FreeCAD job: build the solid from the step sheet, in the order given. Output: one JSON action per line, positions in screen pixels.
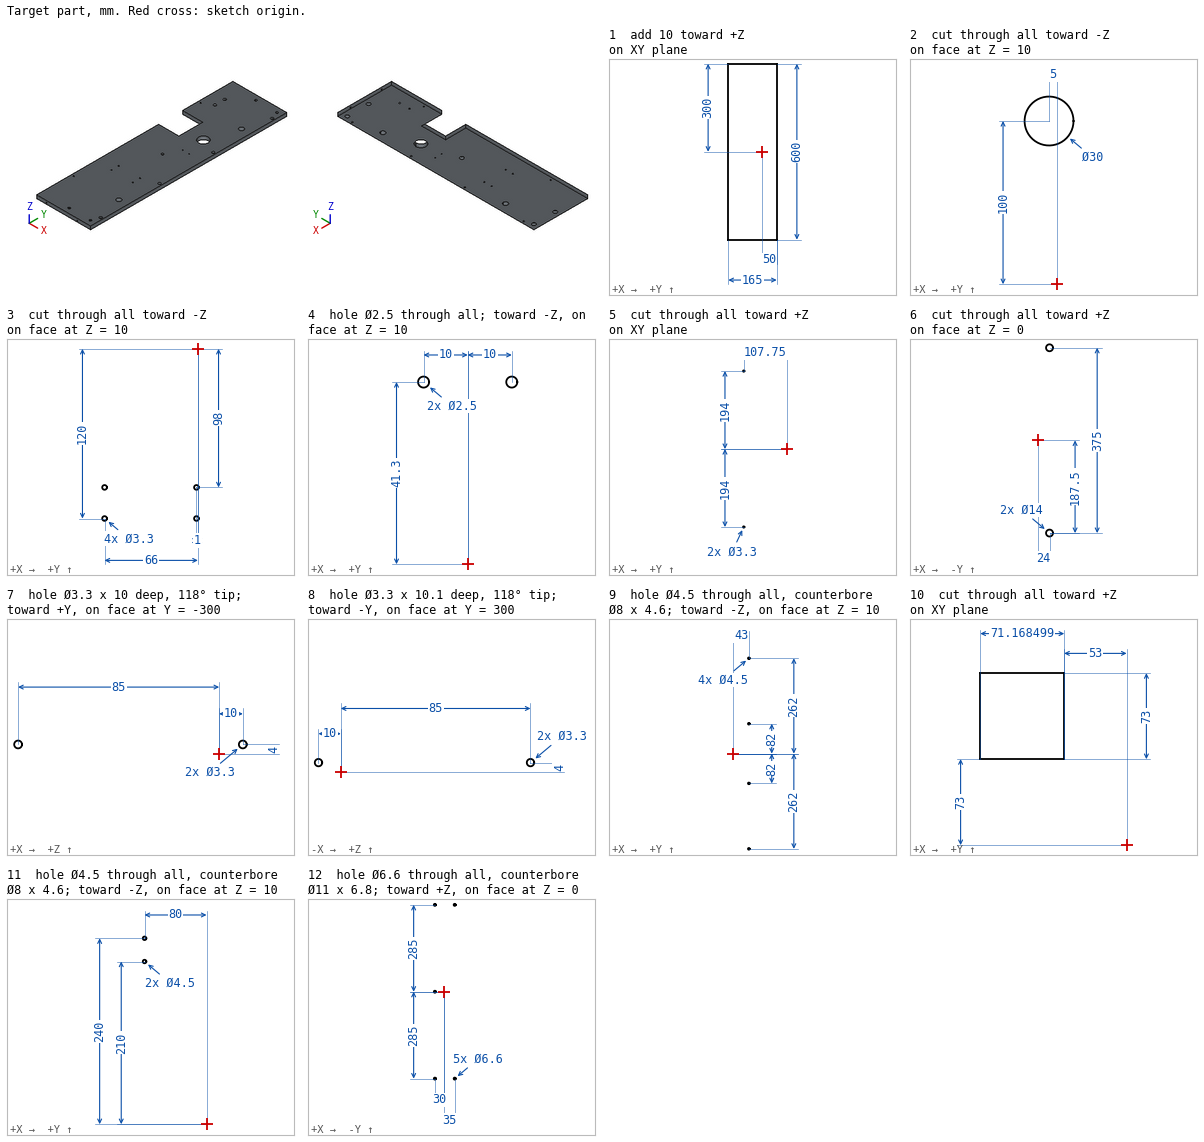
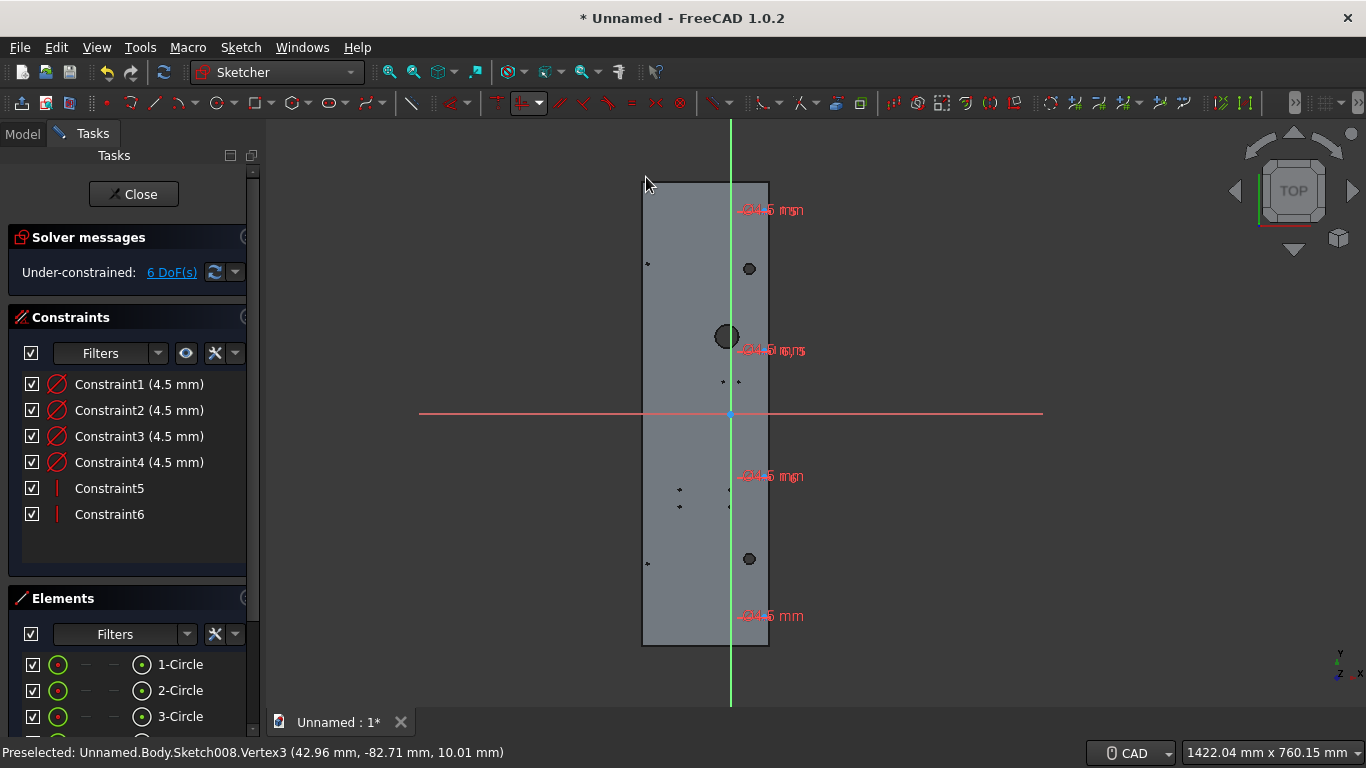
{"action": "left_click", "coordinate": [764, 478]}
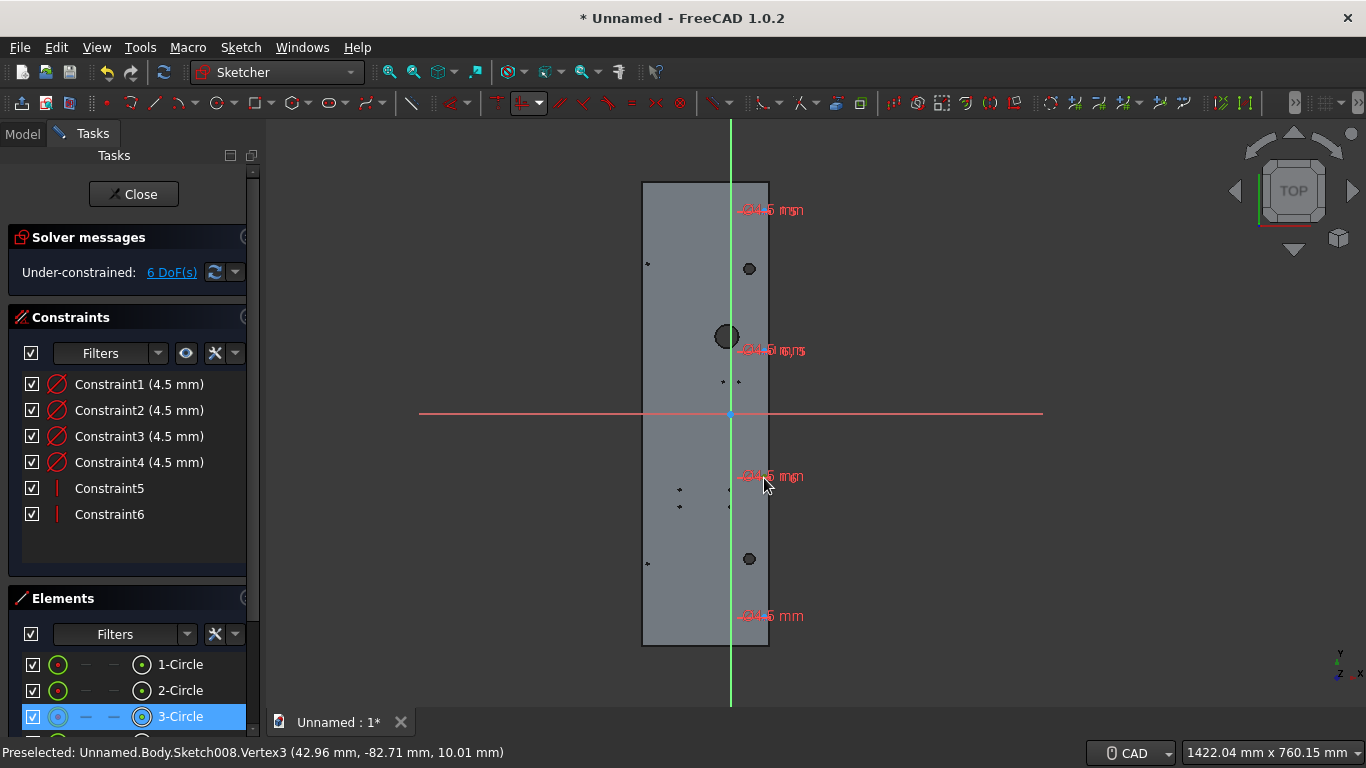
{"action": "left_click", "coordinate": [764, 618]}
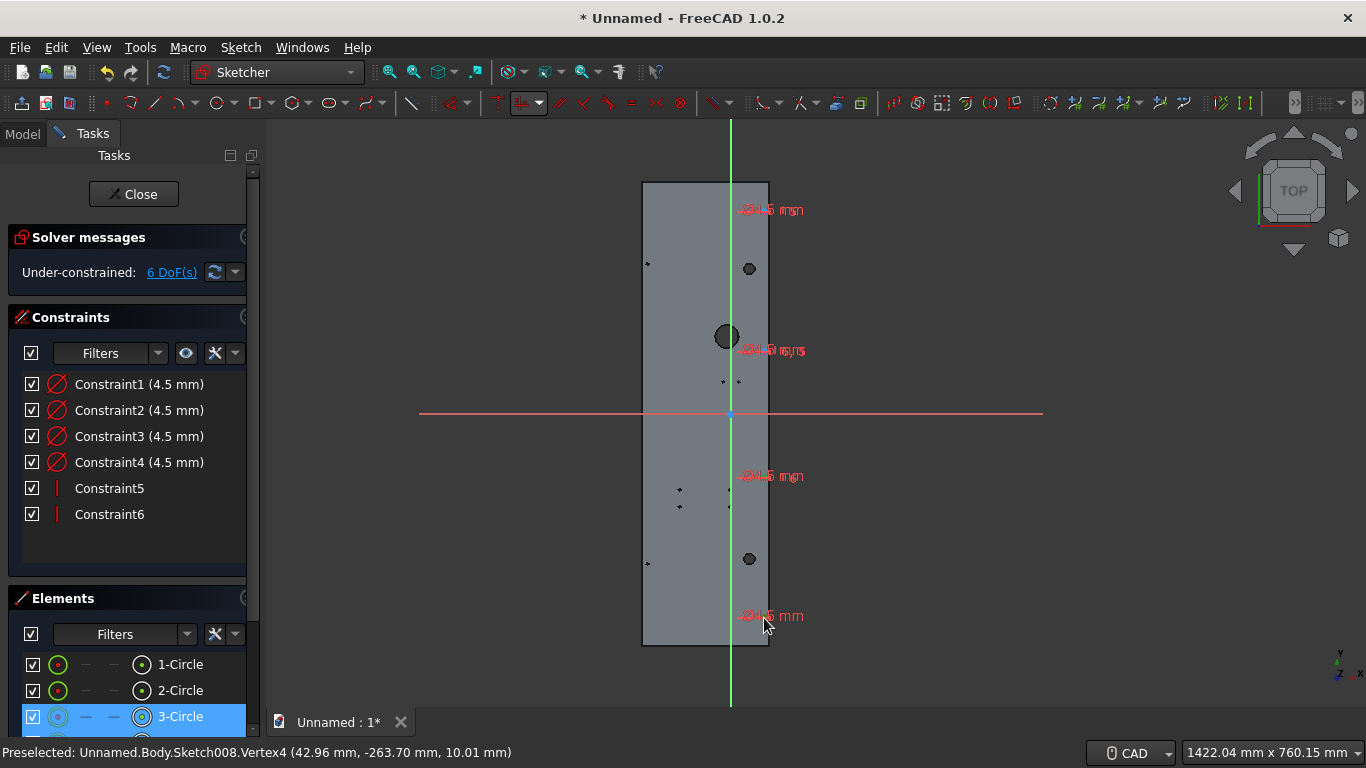
{"action": "left_click", "coordinate": [542, 104]}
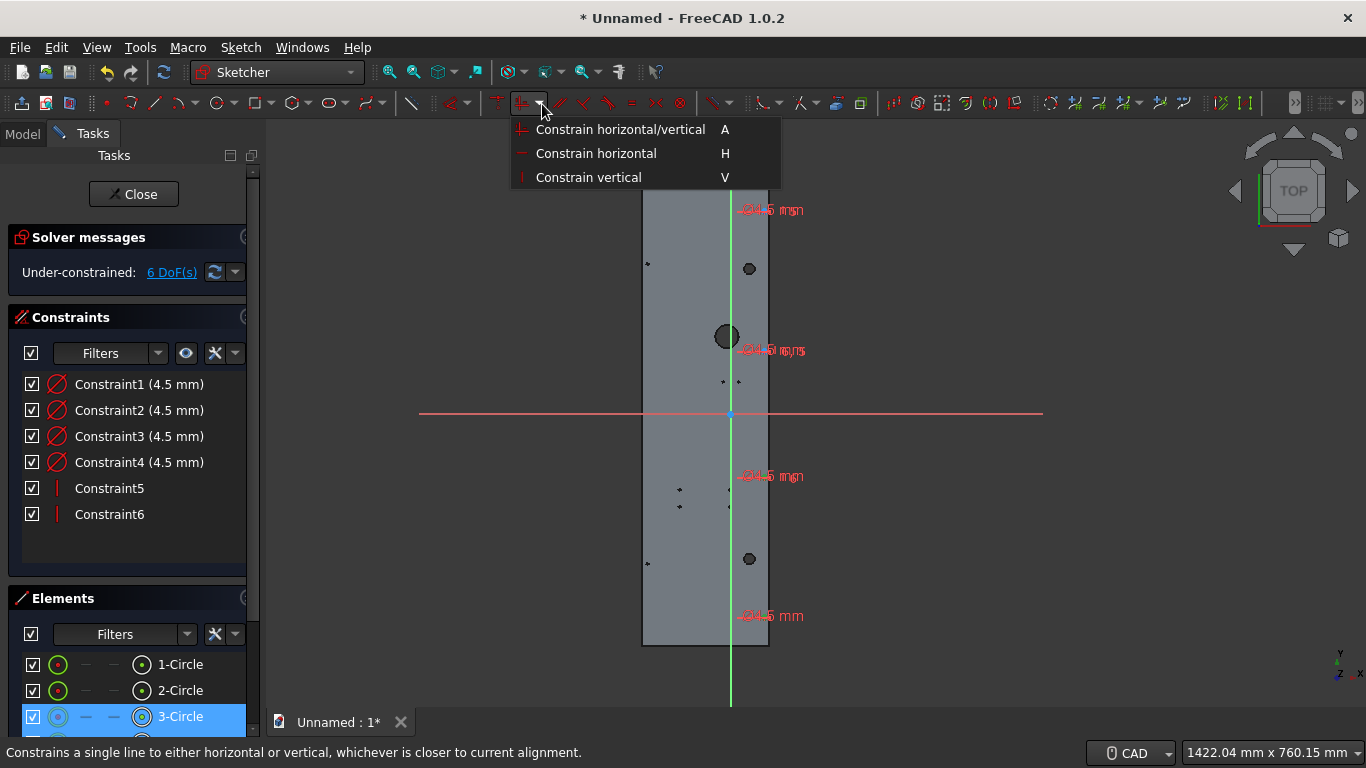
{"action": "left_click", "coordinate": [646, 177]}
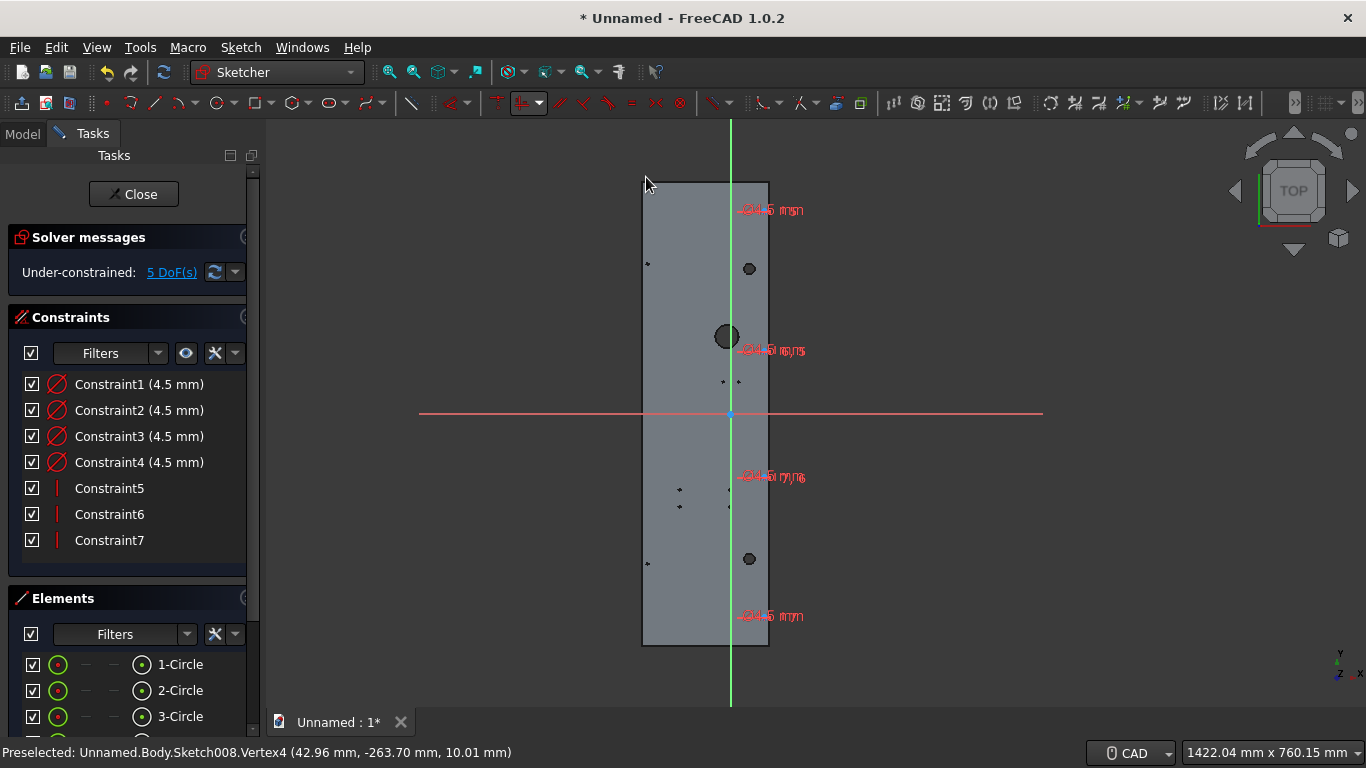
{"action": "left_click", "coordinate": [450, 104]}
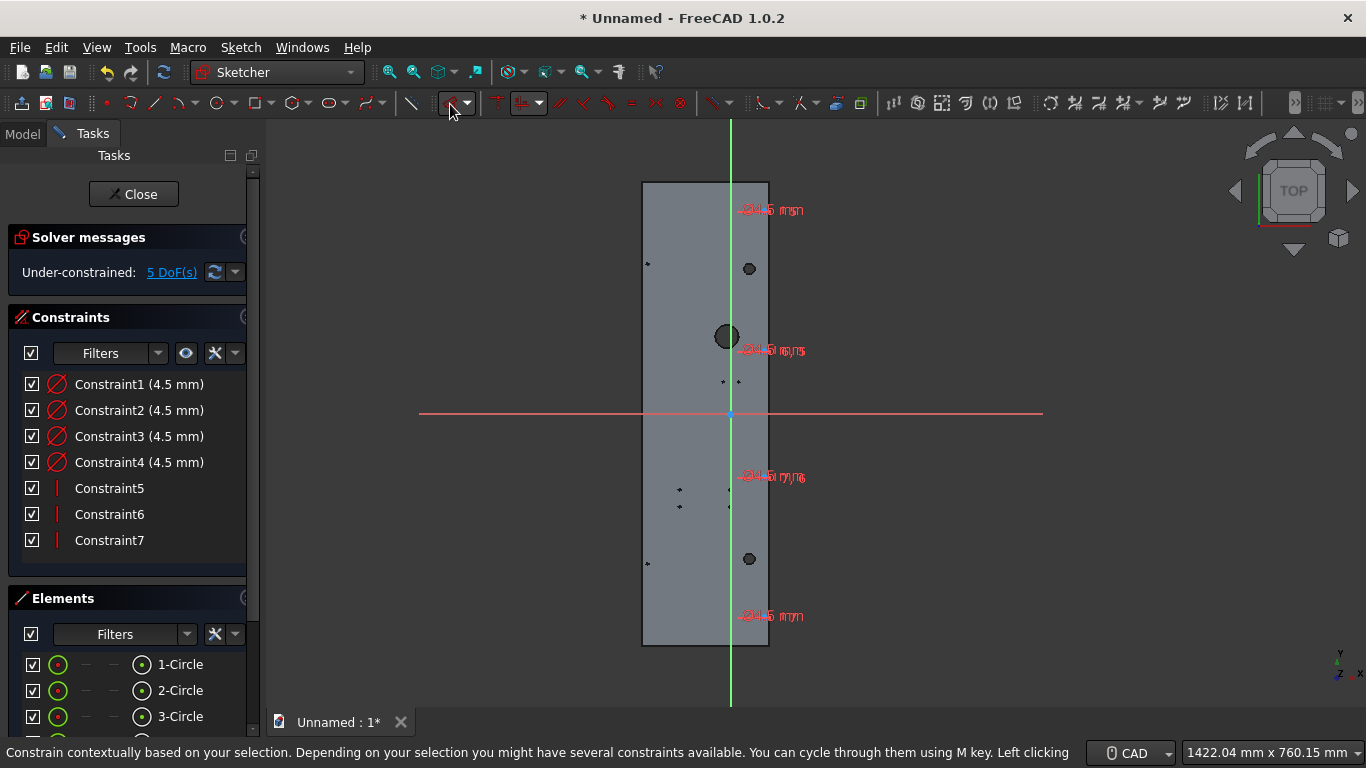
{"action": "left_click", "coordinate": [764, 212]}
{"action": "left_click", "coordinate": [747, 178]}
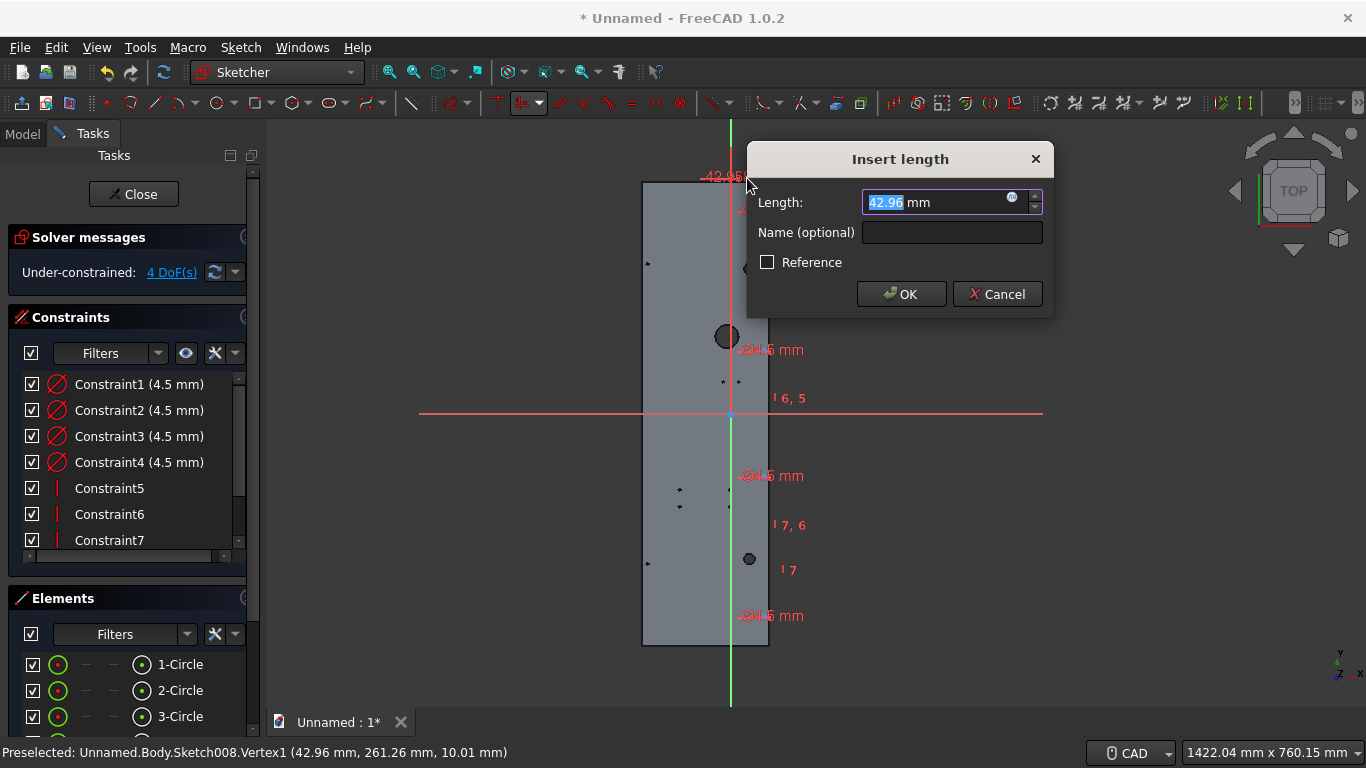
{"action": "type", "text": "43"}
{"action": "key", "text": "Return"}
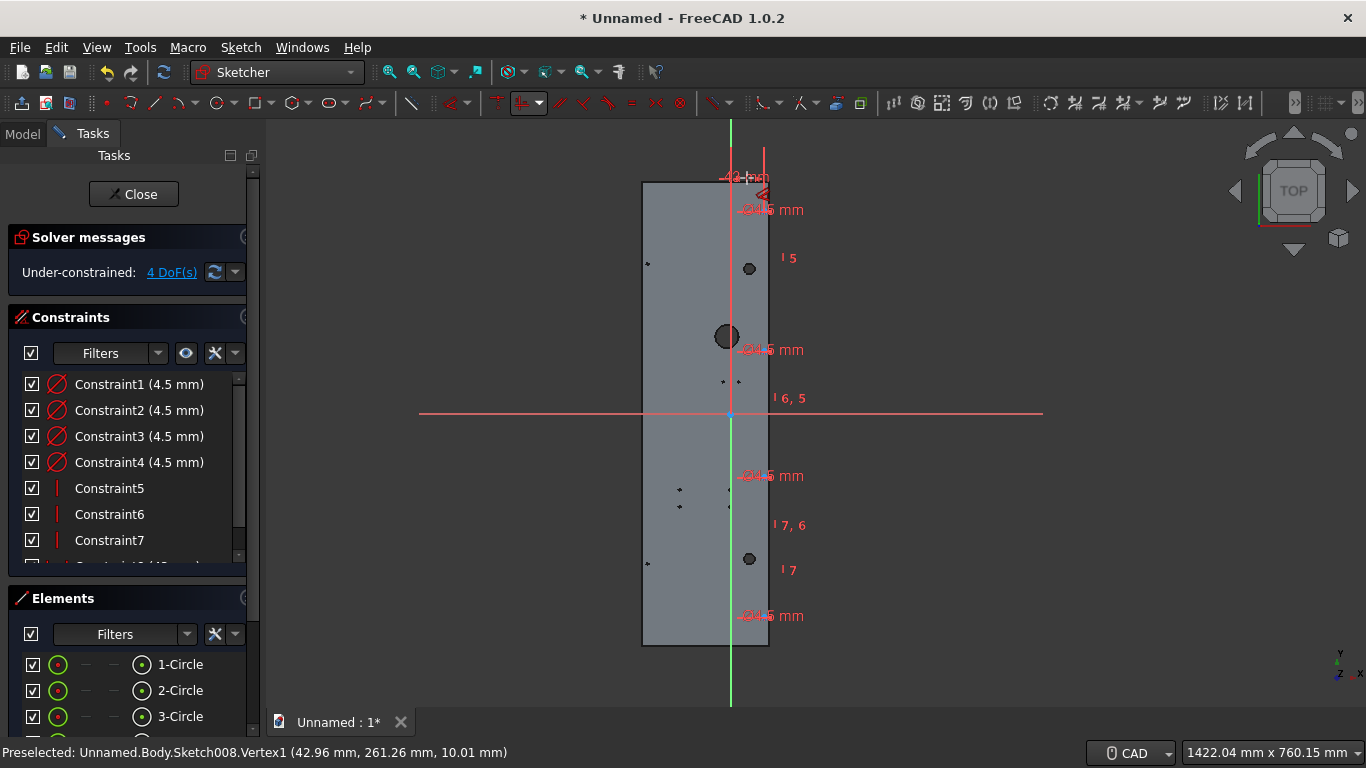
{"action": "left_click", "coordinate": [764, 352]}
{"action": "left_click", "coordinate": [697, 383]}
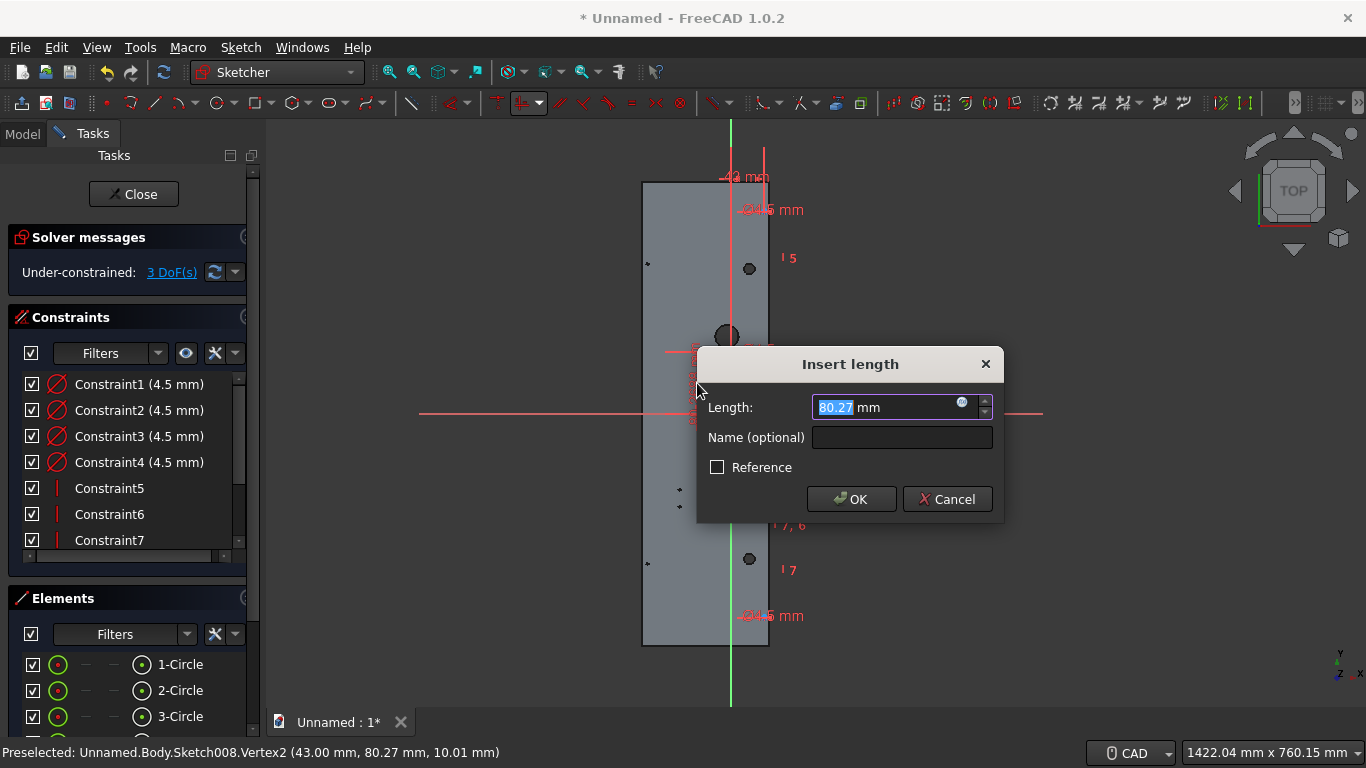
{"action": "type", "text": "82"}
{"action": "key", "text": "Return"}